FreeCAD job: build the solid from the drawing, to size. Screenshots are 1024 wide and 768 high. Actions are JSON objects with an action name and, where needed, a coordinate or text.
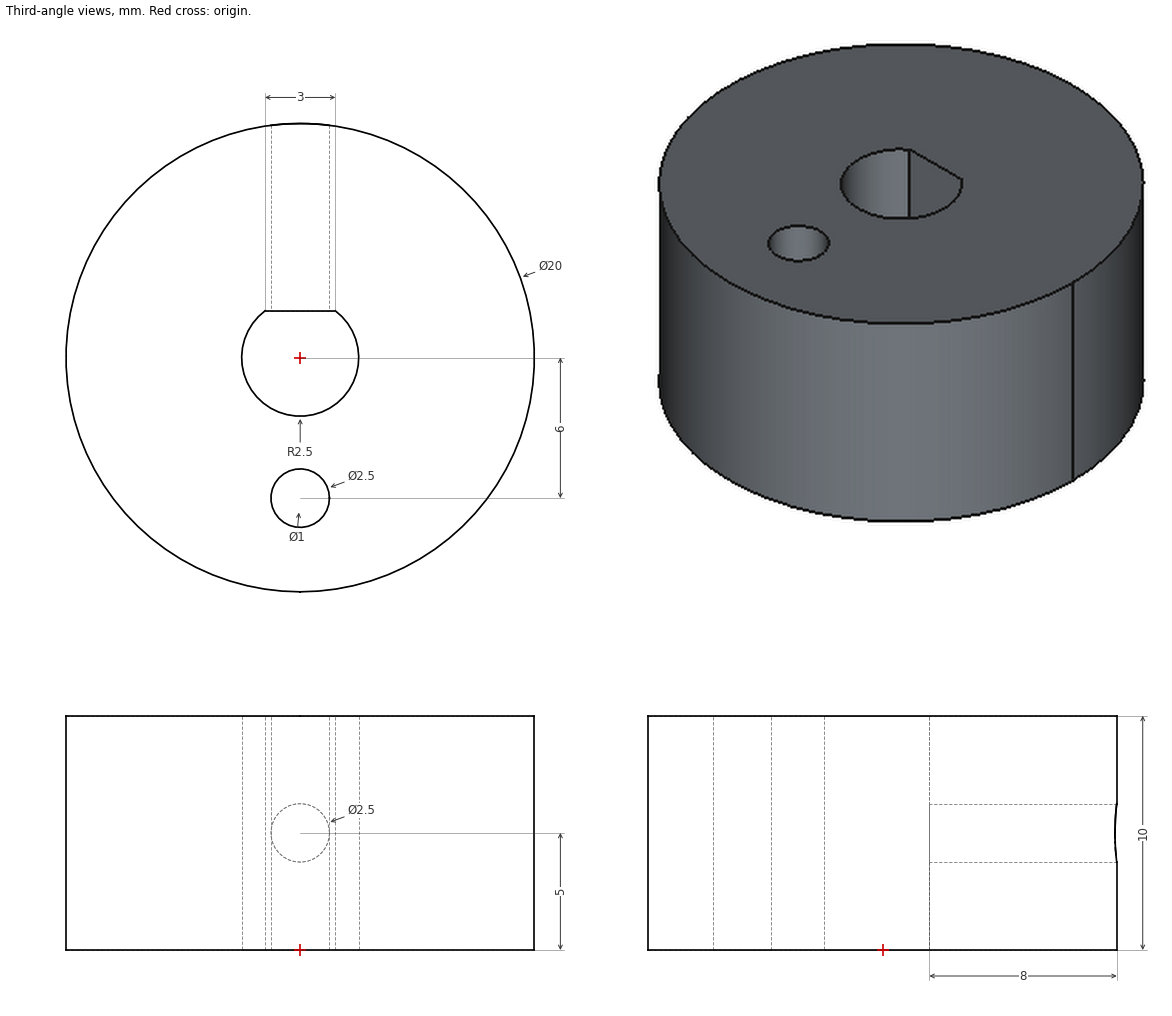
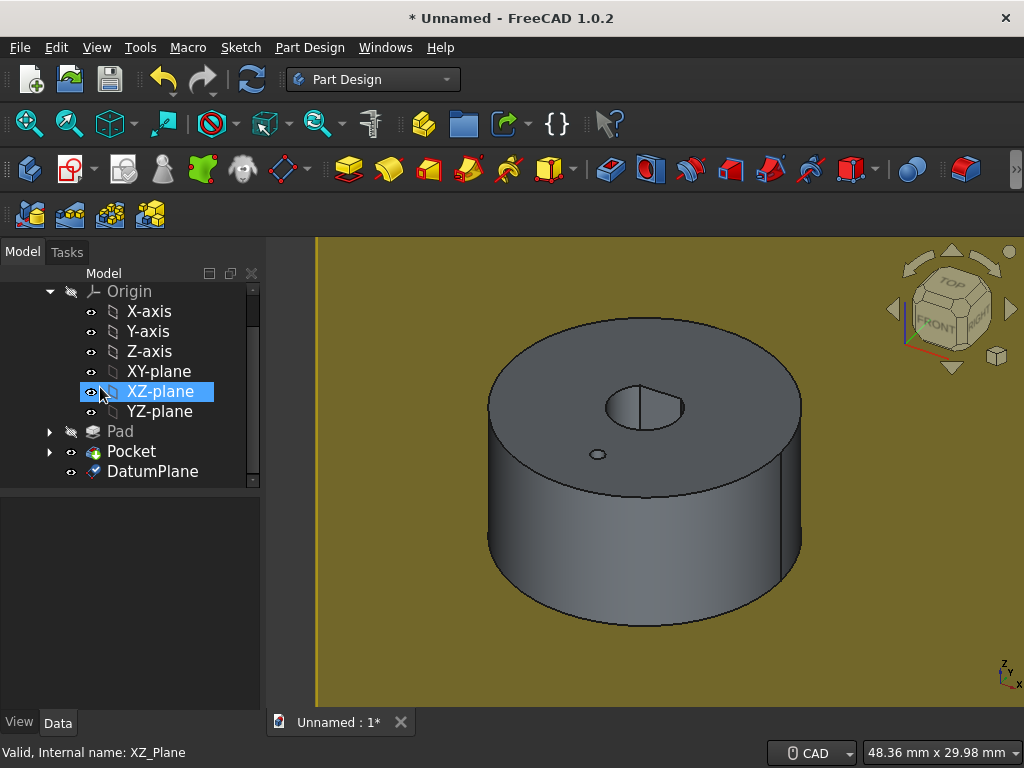
{"action": "left_click", "coordinate": [116, 472]}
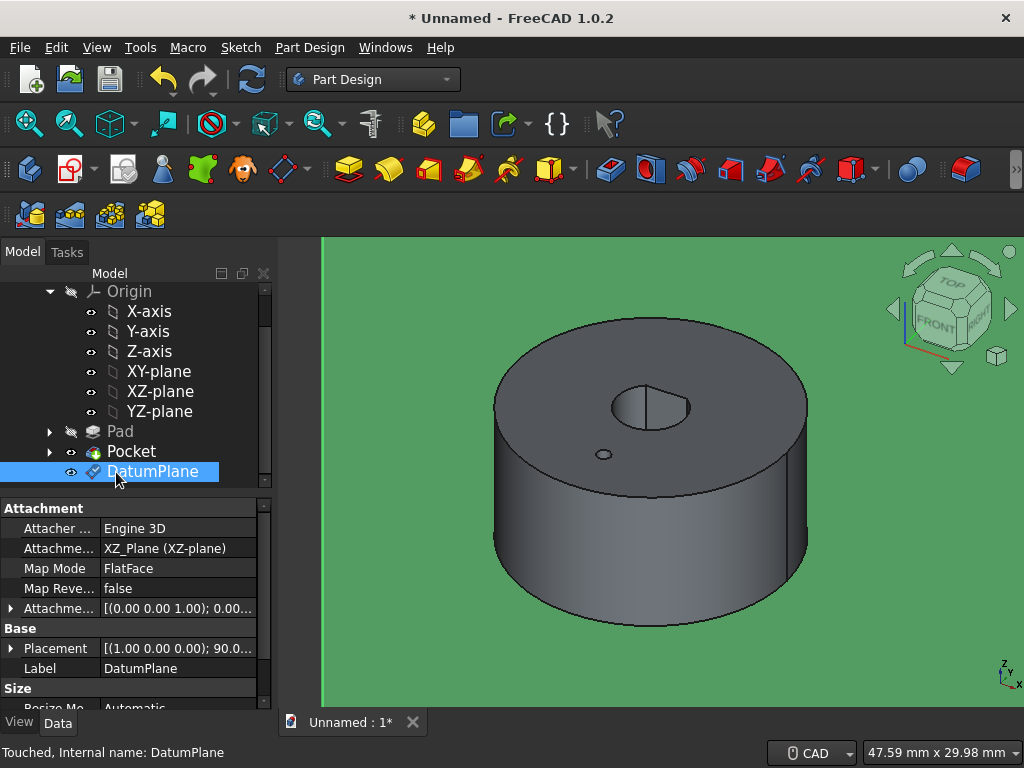
{"action": "left_click", "coordinate": [70, 170]}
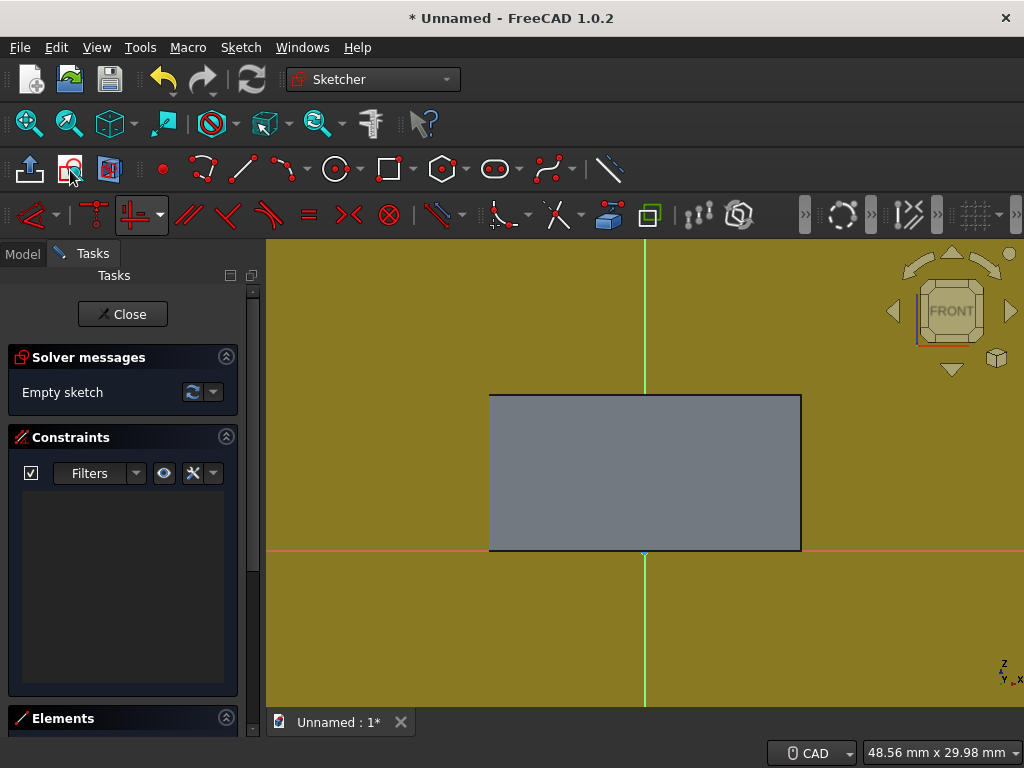
{"action": "key", "text": "q s"}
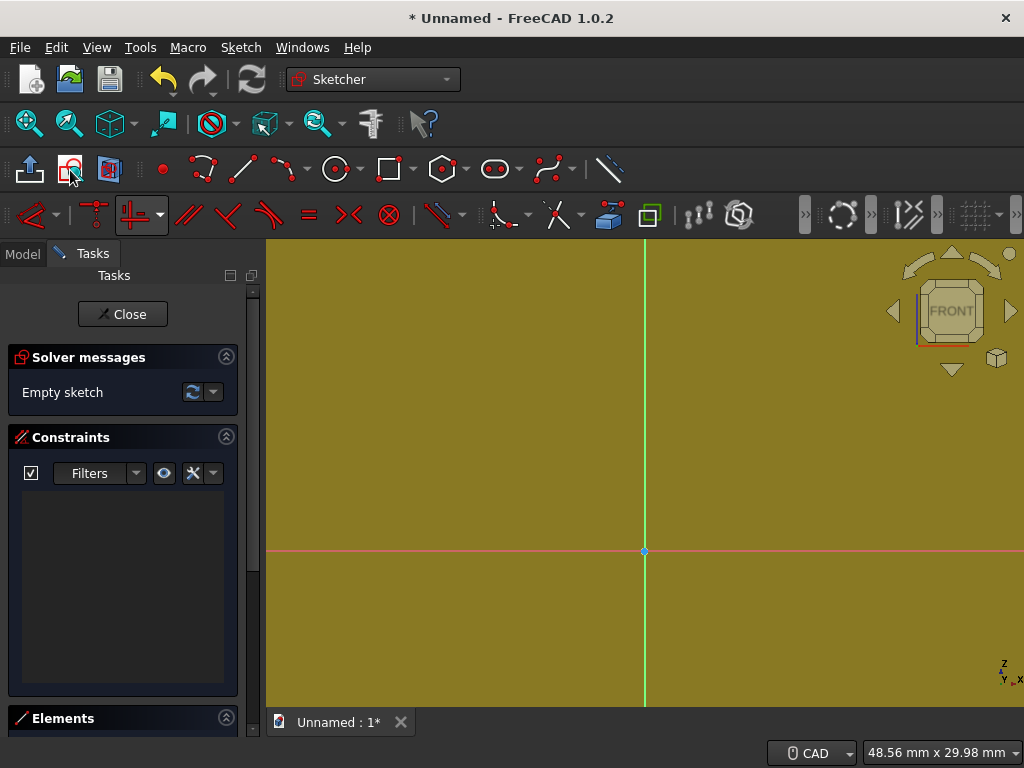
{"action": "scroll", "coordinate": [656, 473], "scroll_direction": "up", "scroll_amount": 10}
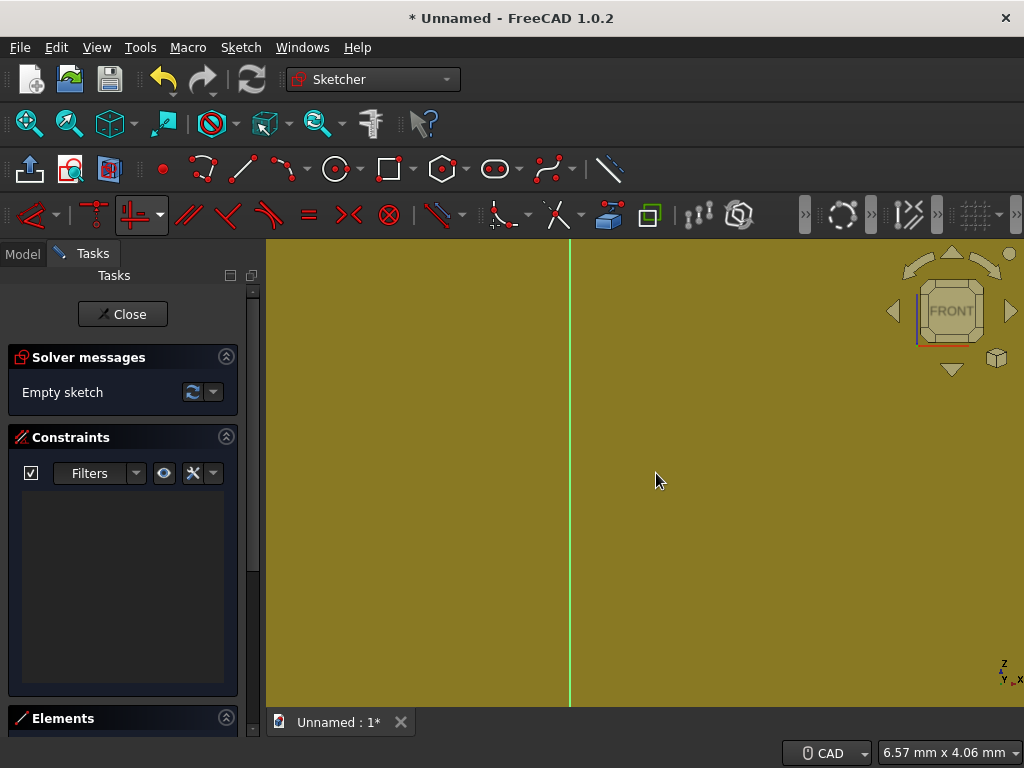
{"action": "key", "text": "g c"}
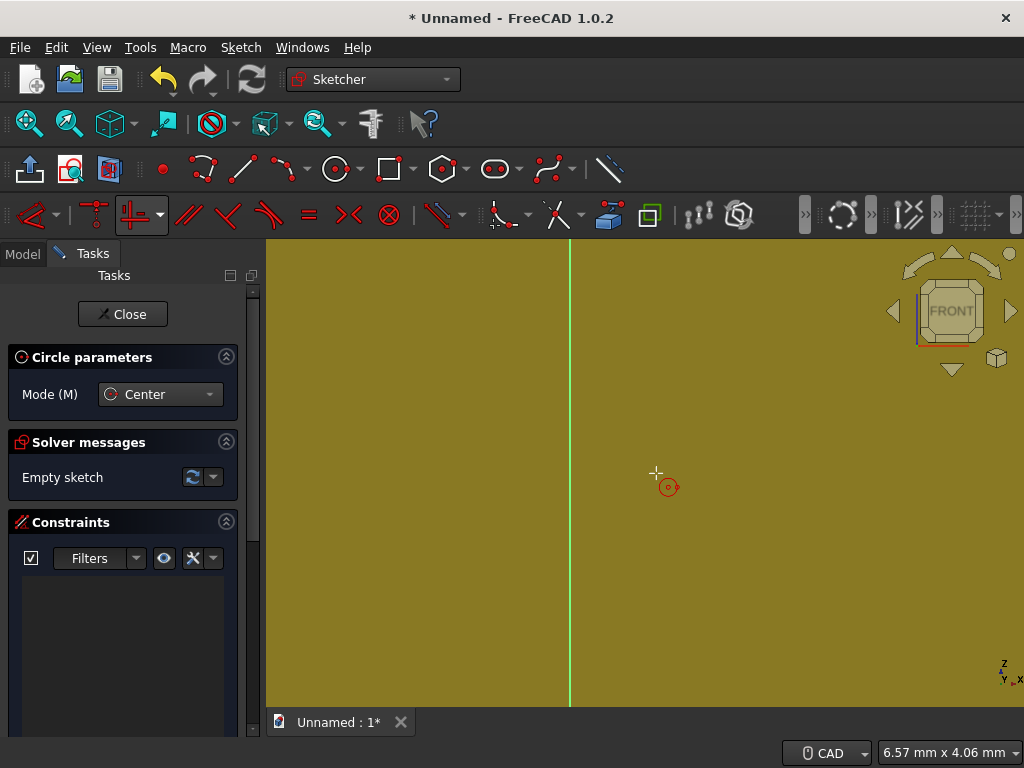
{"action": "left_click", "coordinate": [570, 470]}
{"action": "mouse_move", "coordinate": [672, 368]}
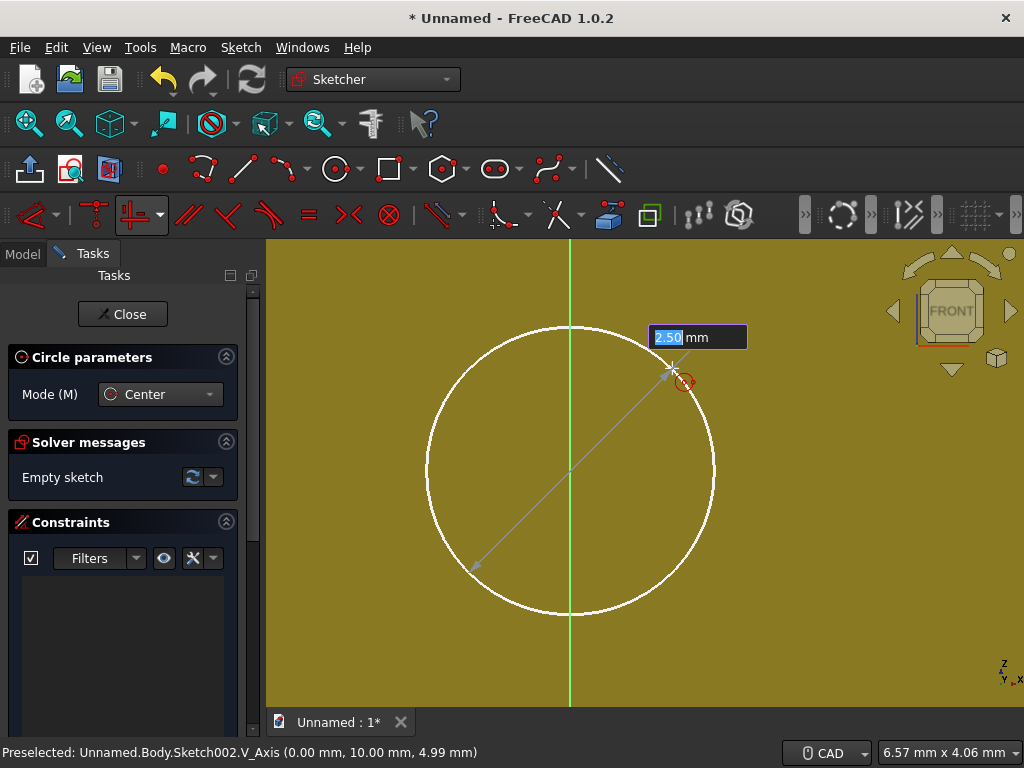
{"action": "type", "text": "2.5"}
{"action": "key", "text": "Return"}
{"action": "key", "text": "Escape"}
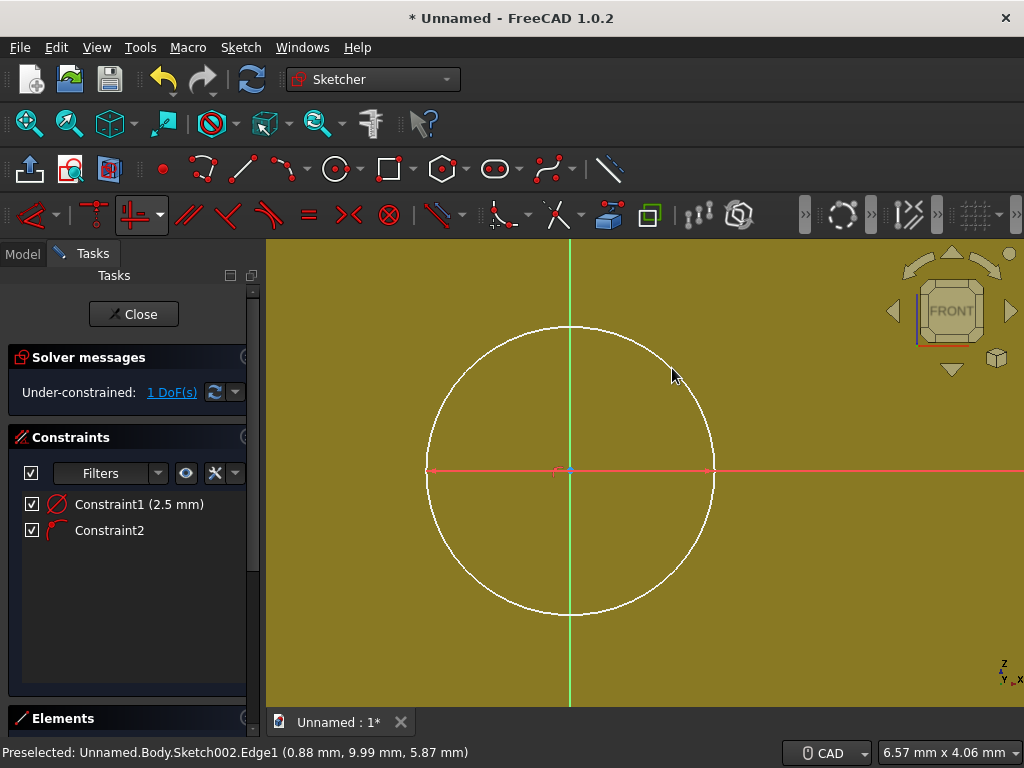
{"action": "key", "text": "d"}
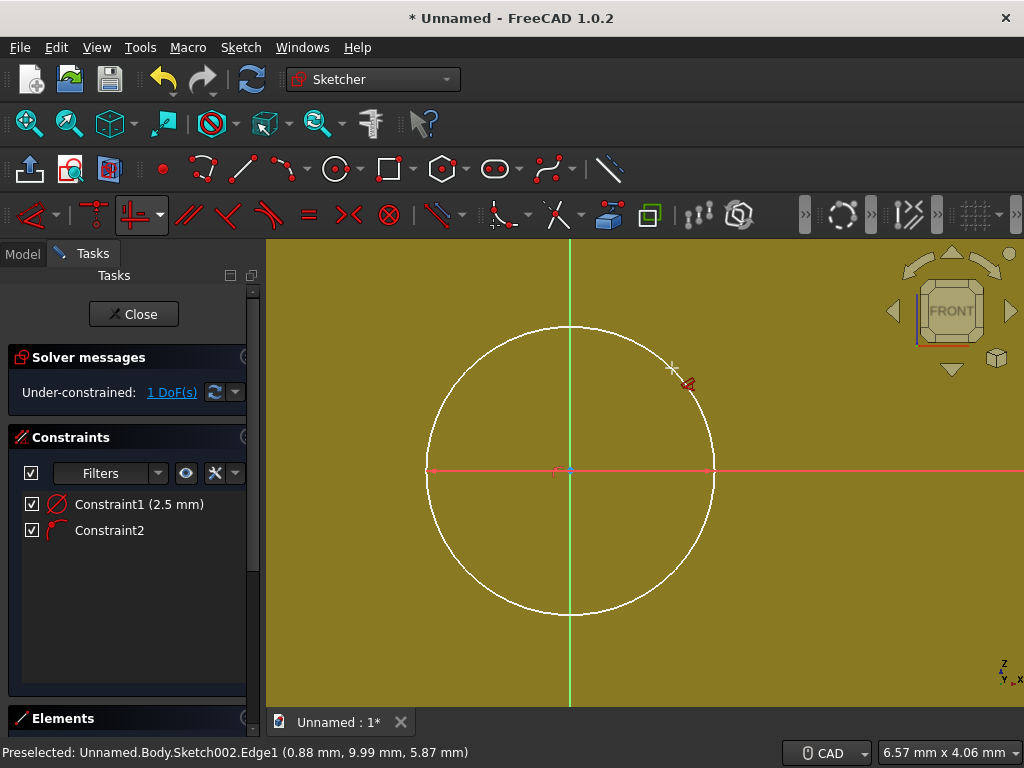
{"action": "left_click", "coordinate": [570, 471]}
{"action": "left_click", "coordinate": [604, 575]}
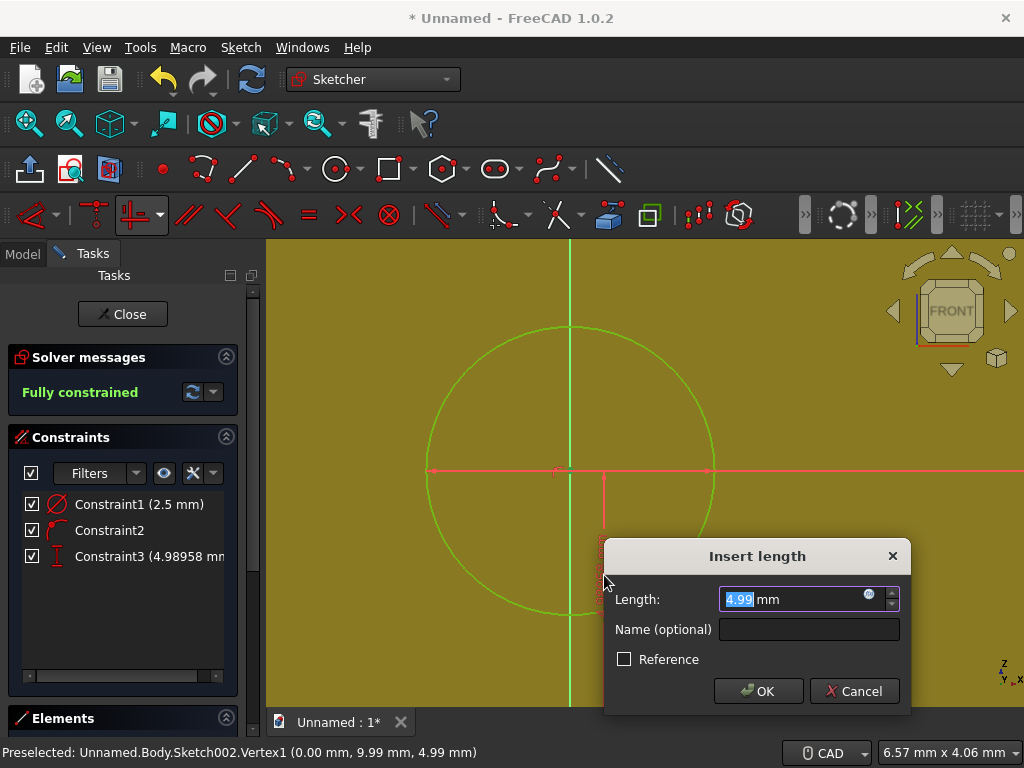
{"action": "type", "text": "5"}
{"action": "key", "text": "Return"}
{"action": "key", "text": "Escape"}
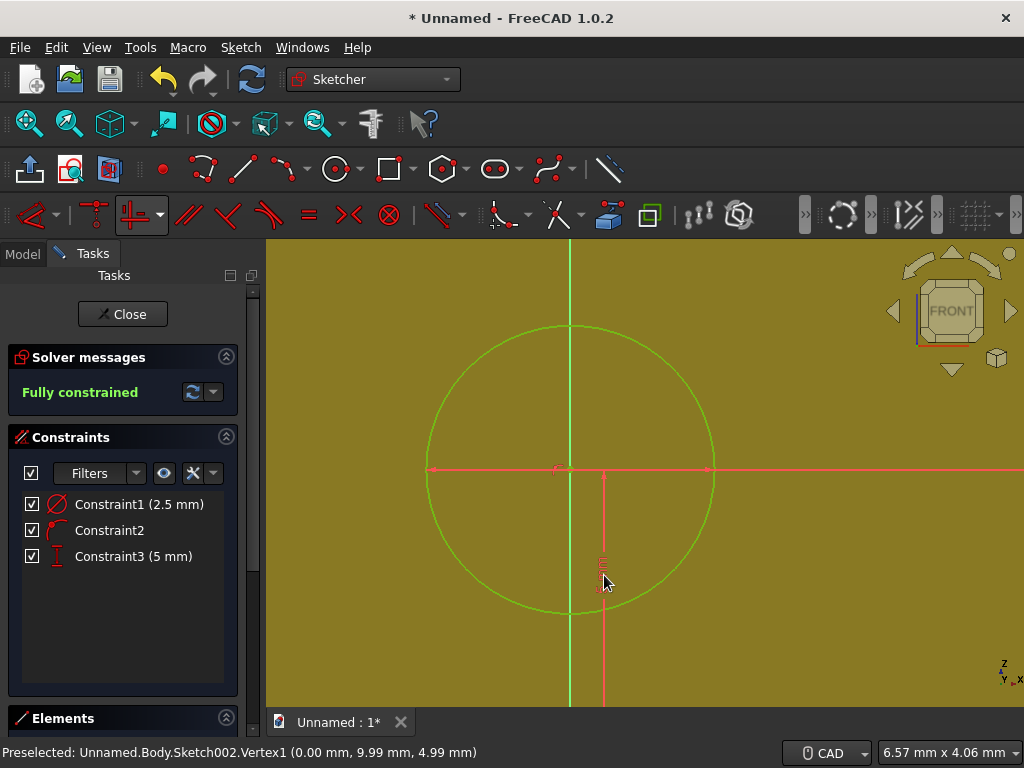
{"action": "left_click", "coordinate": [123, 314]}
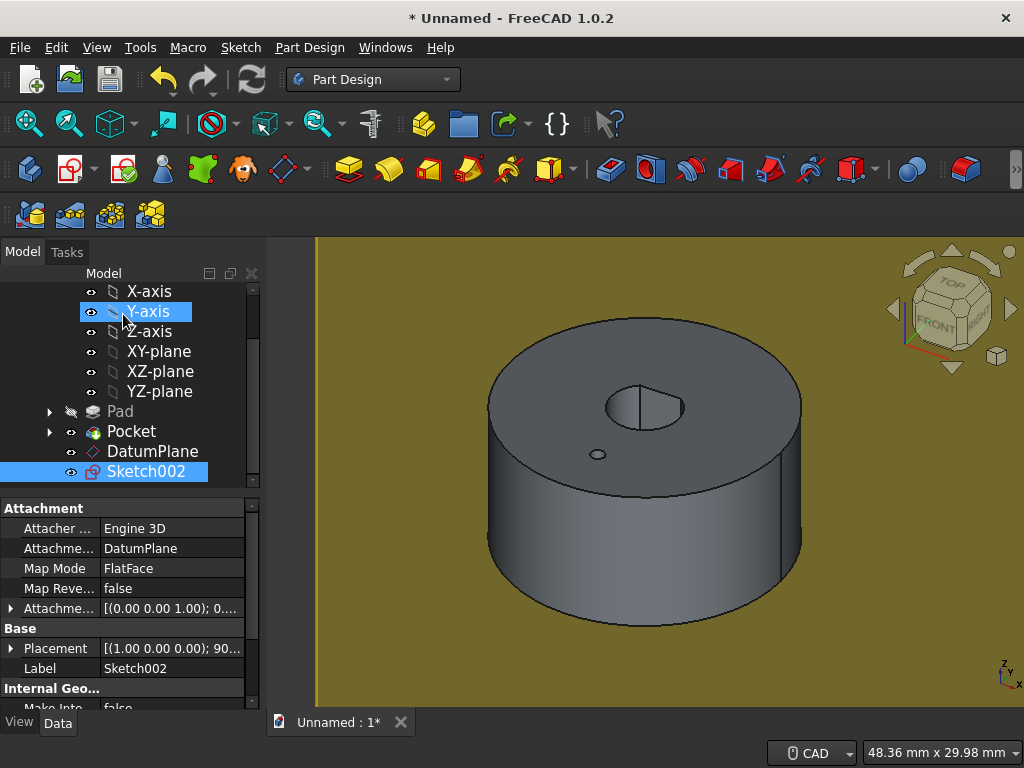
{"action": "left_click", "coordinate": [612, 170]}